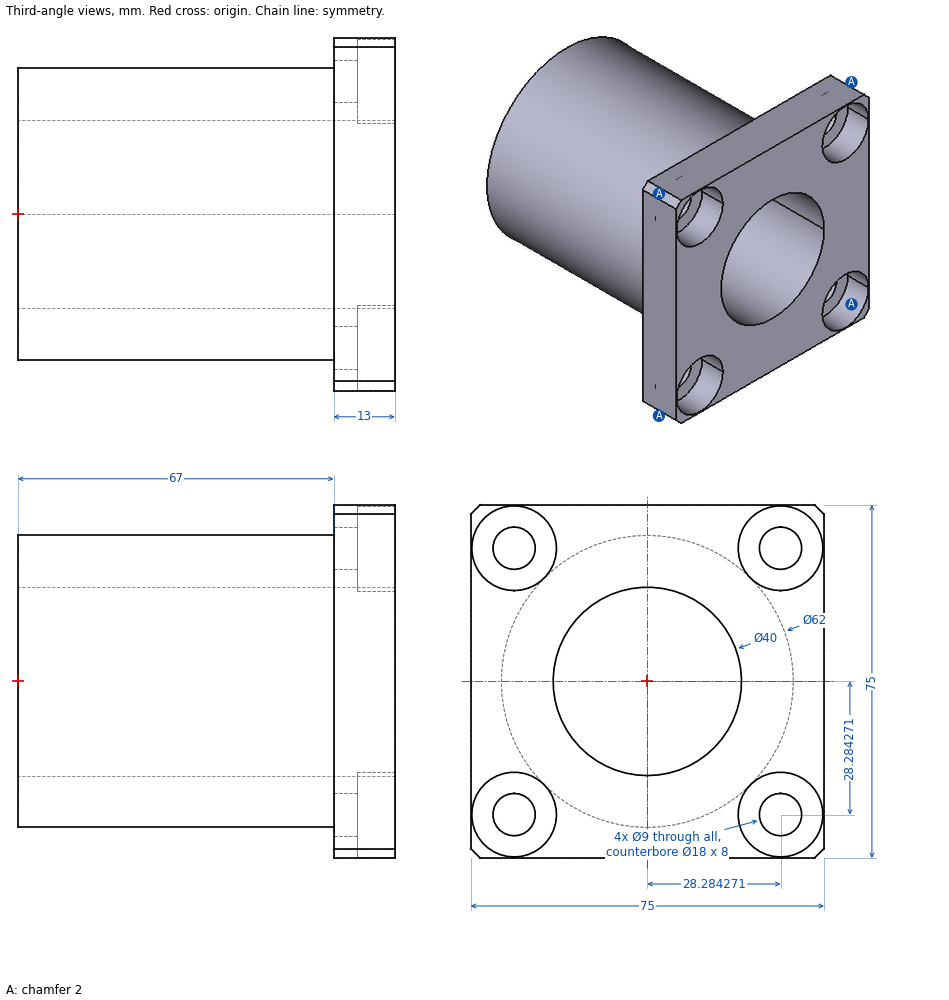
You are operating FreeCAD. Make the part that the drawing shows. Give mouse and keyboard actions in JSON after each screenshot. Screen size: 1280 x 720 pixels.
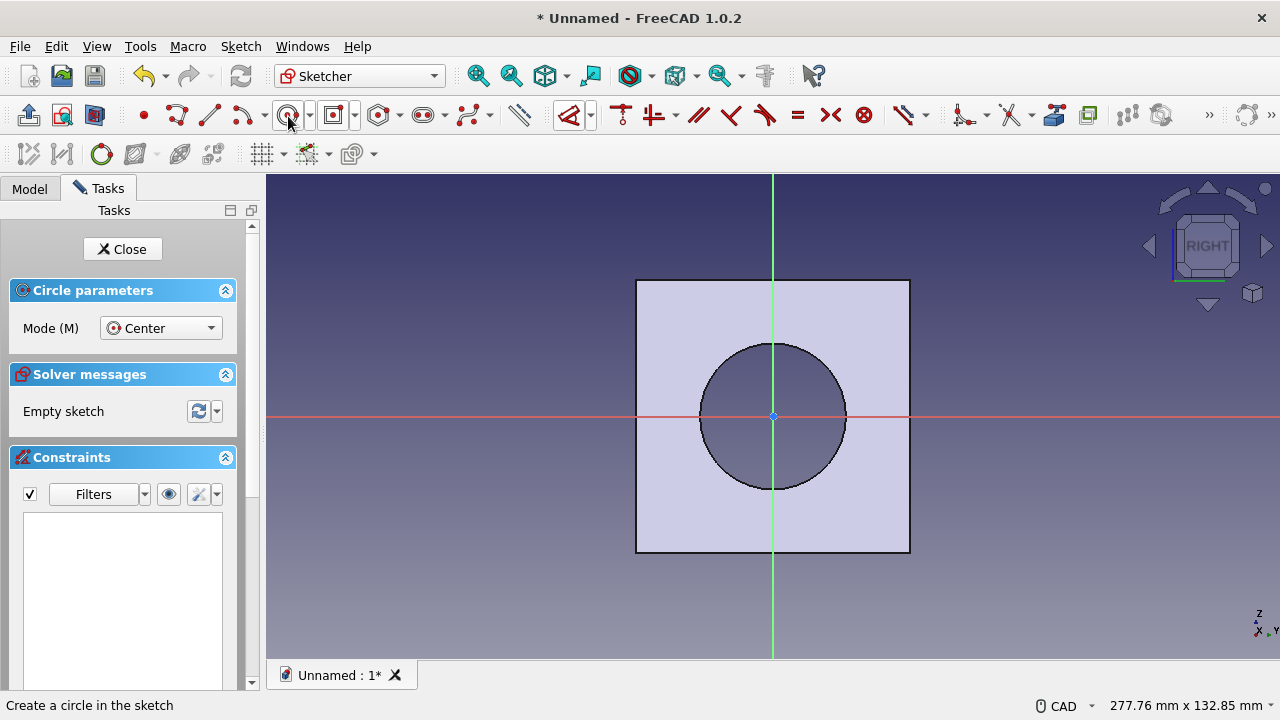
{"action": "scroll", "coordinate": [876, 520], "scroll_direction": "up", "scroll_amount": 2}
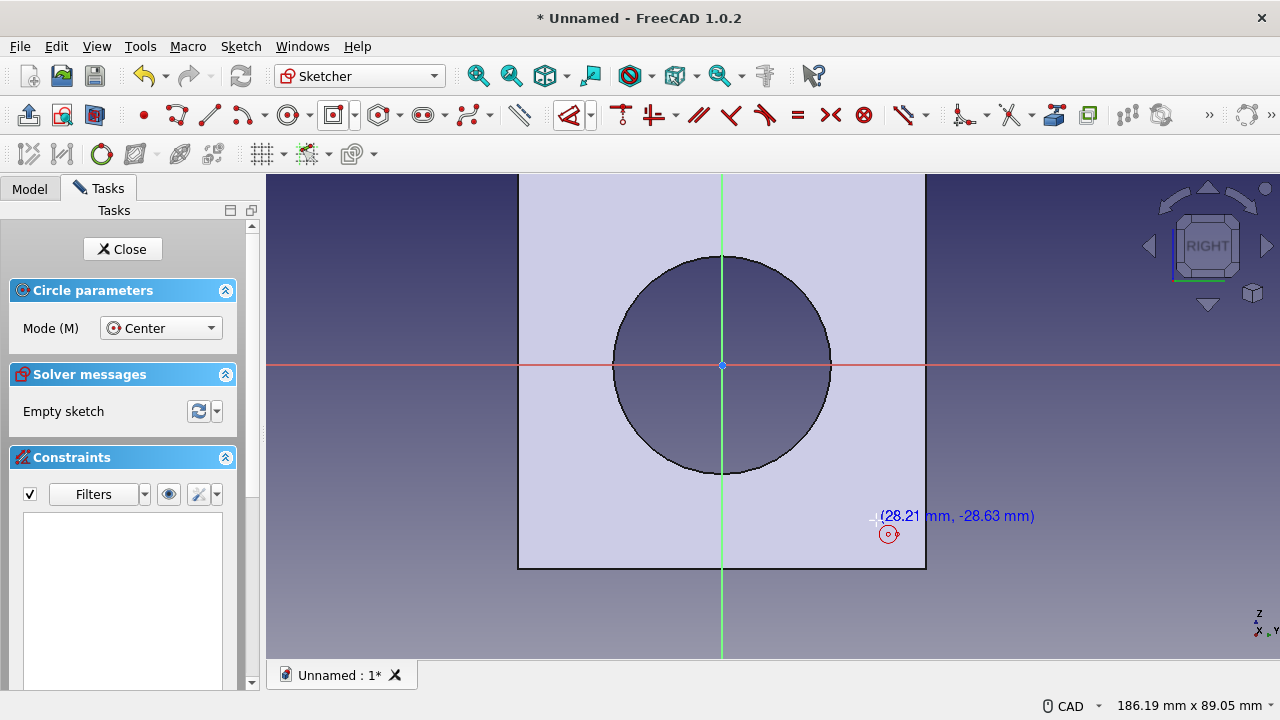
{"action": "left_click", "coordinate": [876, 519]}
{"action": "left_click", "coordinate": [893, 502]}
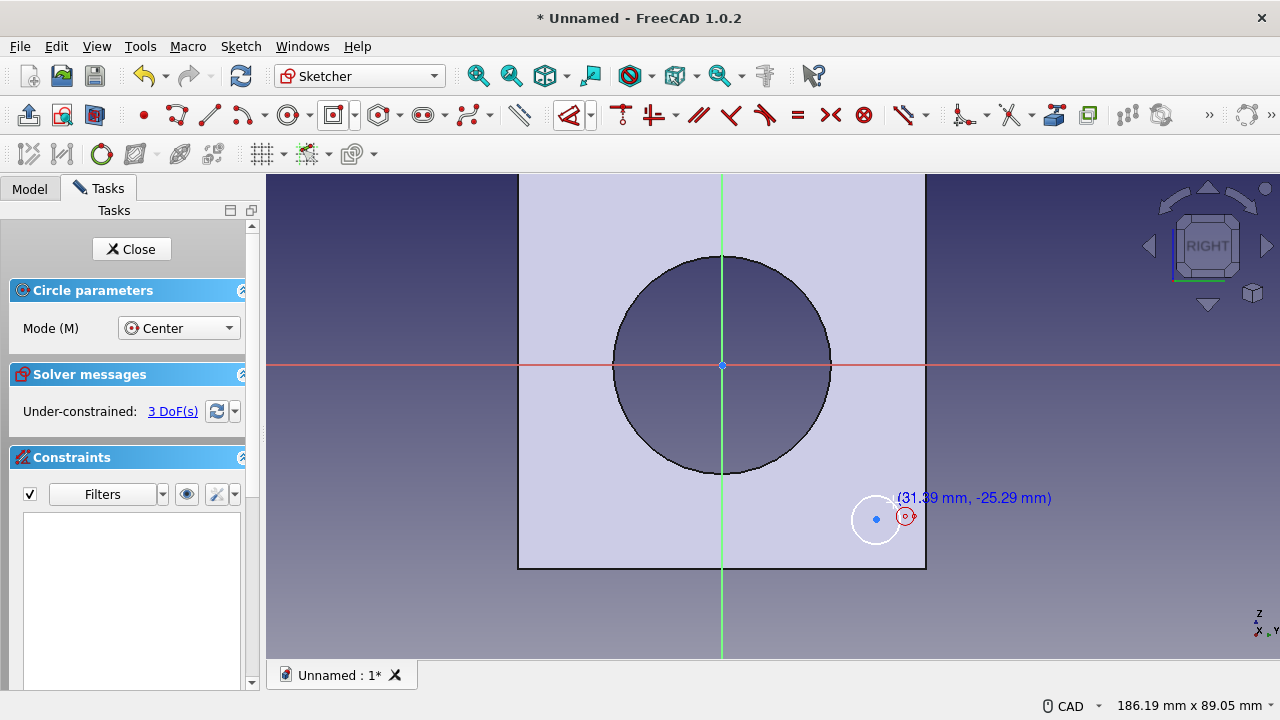
{"action": "left_click", "coordinate": [568, 519]}
{"action": "left_click", "coordinate": [585, 502]}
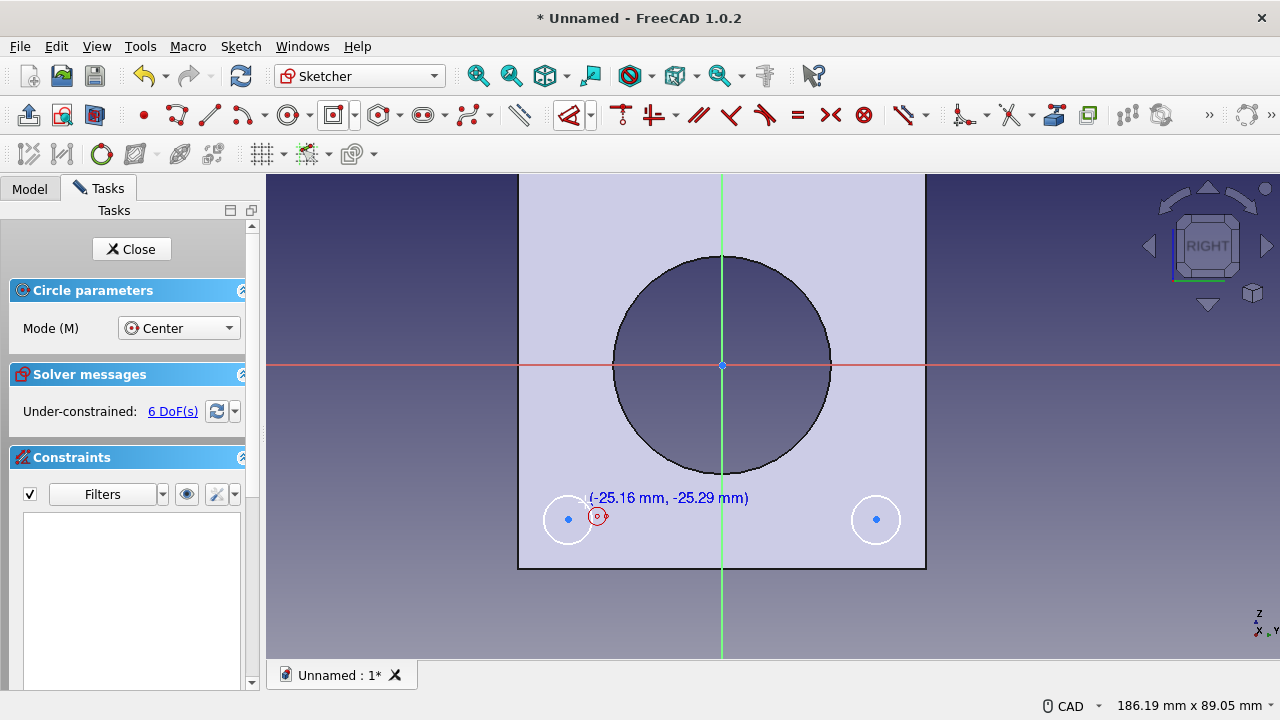
{"action": "left_click", "coordinate": [568, 211]}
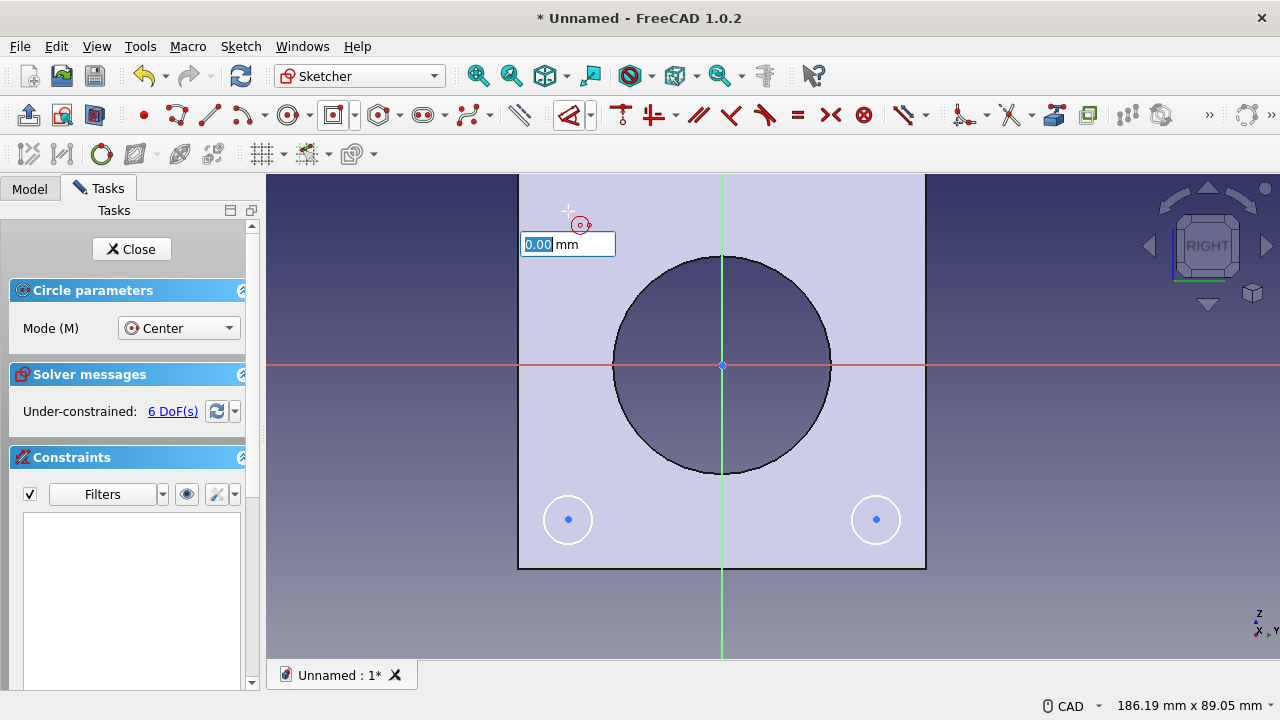
{"action": "scroll", "coordinate": [625, 631], "scroll_direction": "down", "scroll_amount": 1}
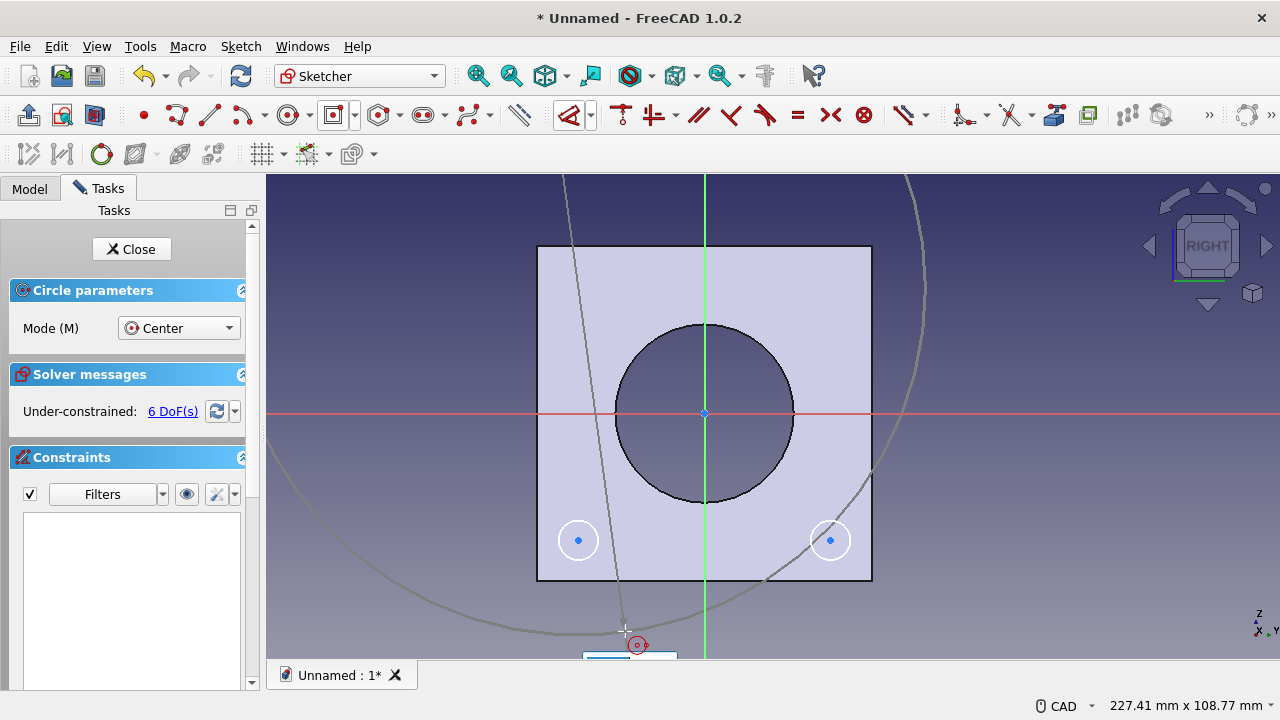
{"action": "left_click", "coordinate": [593, 273]}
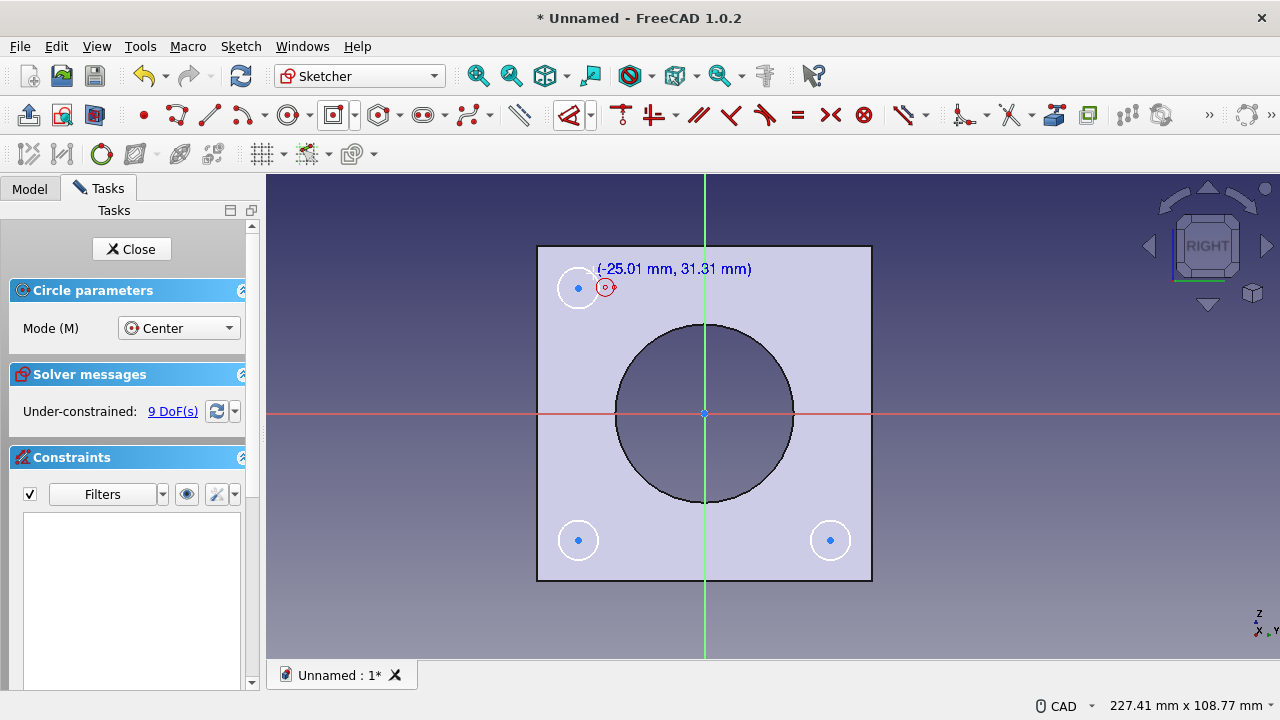
{"action": "left_click", "coordinate": [831, 287]}
{"action": "left_click", "coordinate": [845, 273]}
{"action": "key", "text": "Escape"}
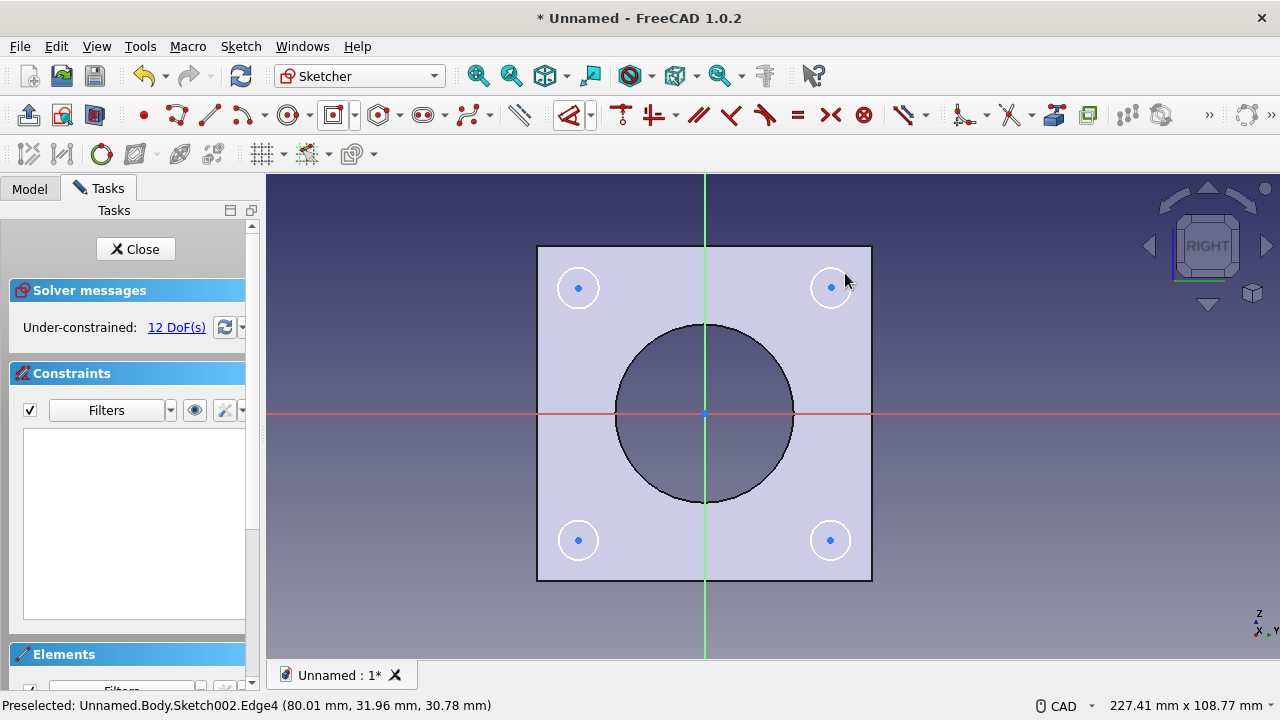
{"action": "left_click", "coordinate": [844, 526]}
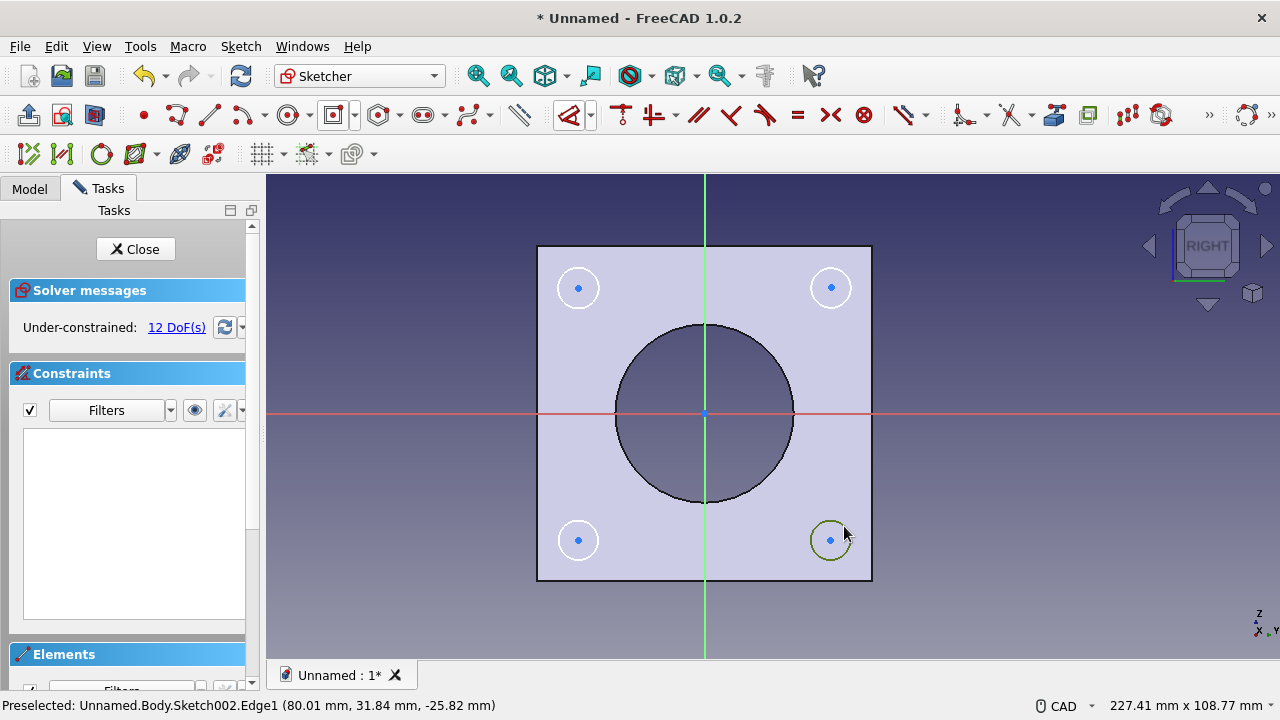
{"action": "left_click", "coordinate": [592, 526]}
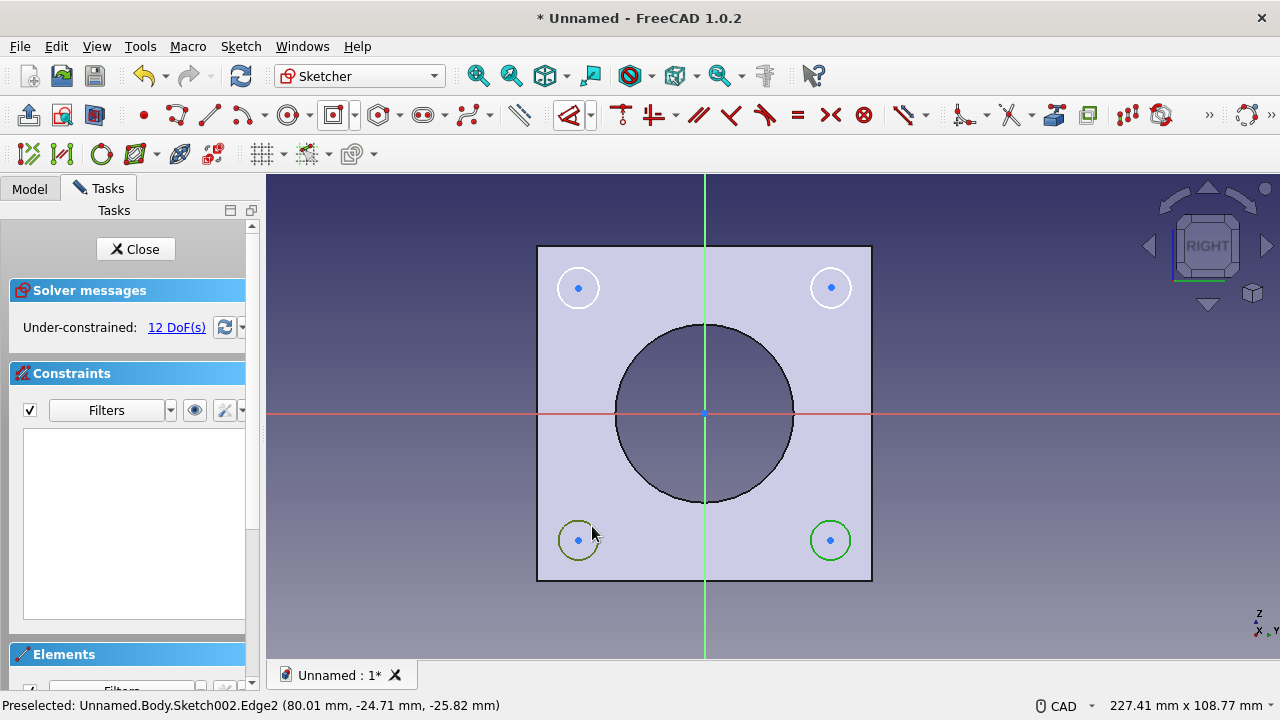
{"action": "left_click", "coordinate": [593, 274]}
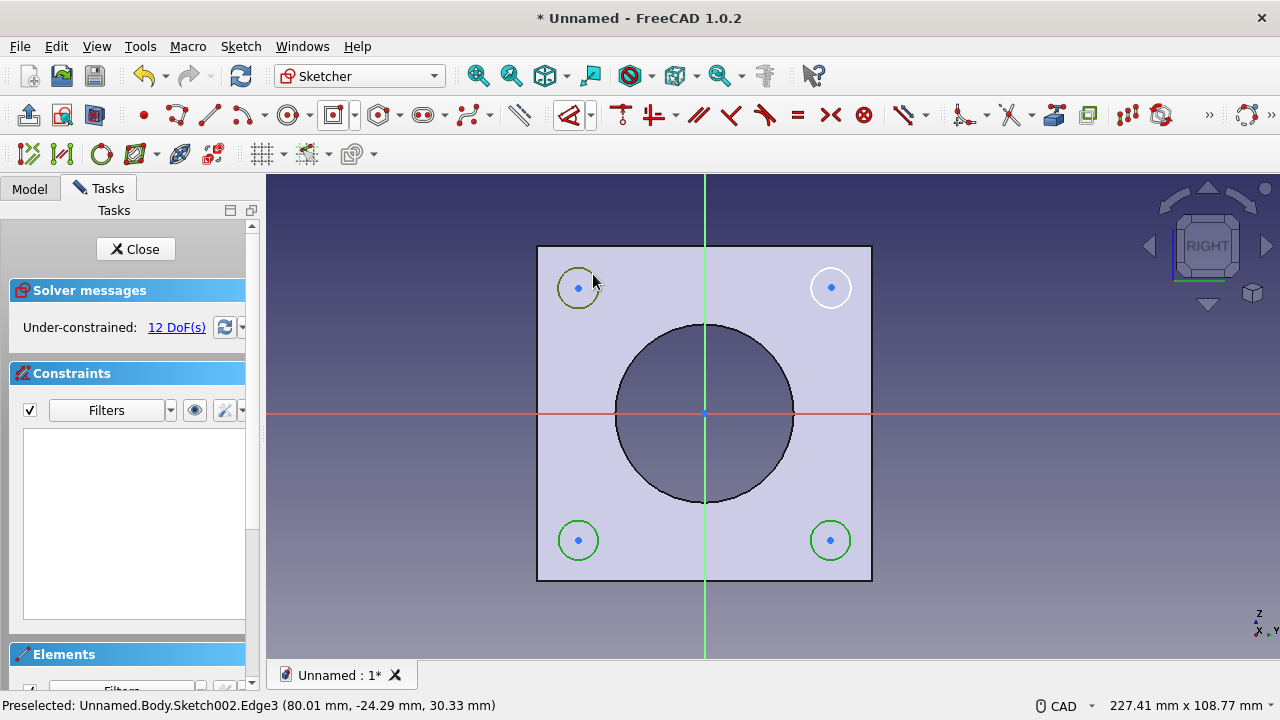
{"action": "left_click", "coordinate": [845, 274]}